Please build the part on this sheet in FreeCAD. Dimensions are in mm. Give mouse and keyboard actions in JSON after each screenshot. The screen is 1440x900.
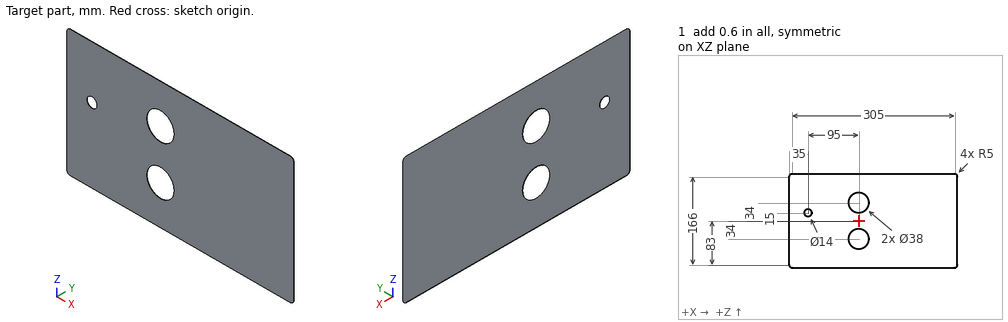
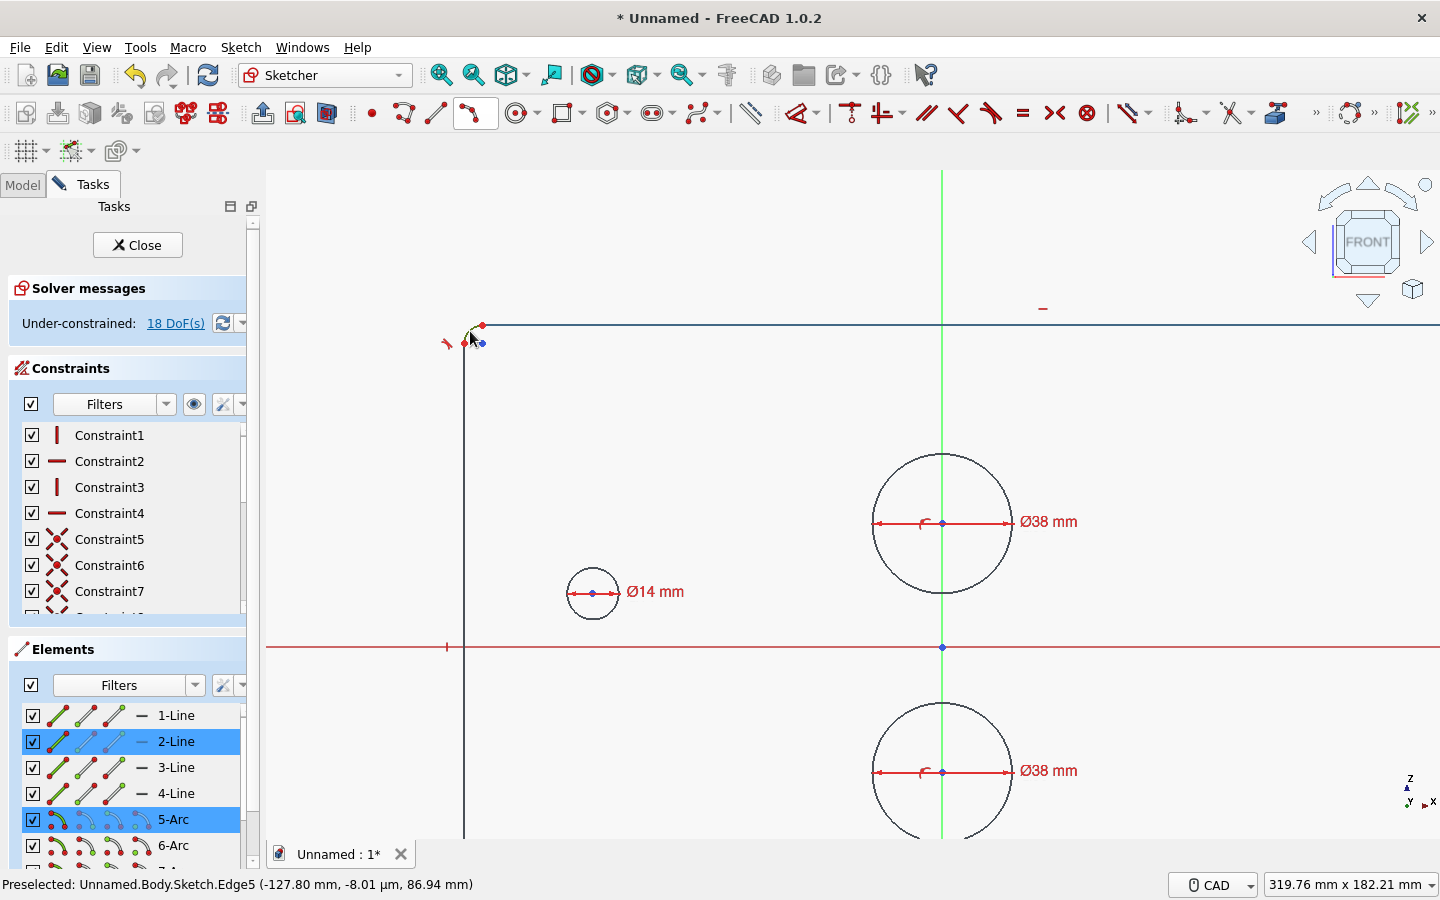
{"action": "left_click", "coordinate": [992, 114]}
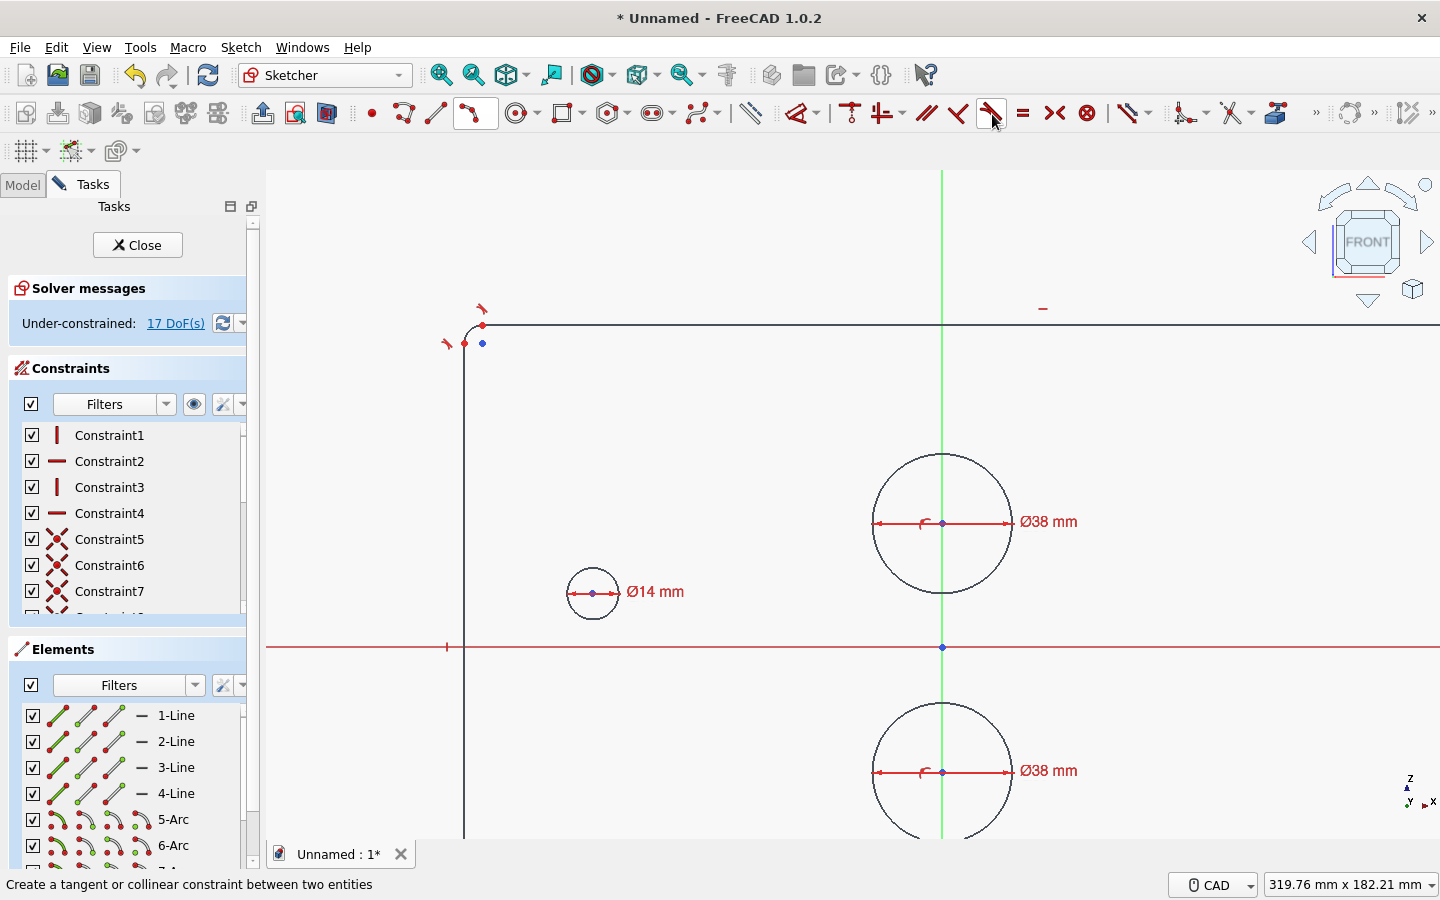
{"action": "left_click", "coordinate": [819, 325]}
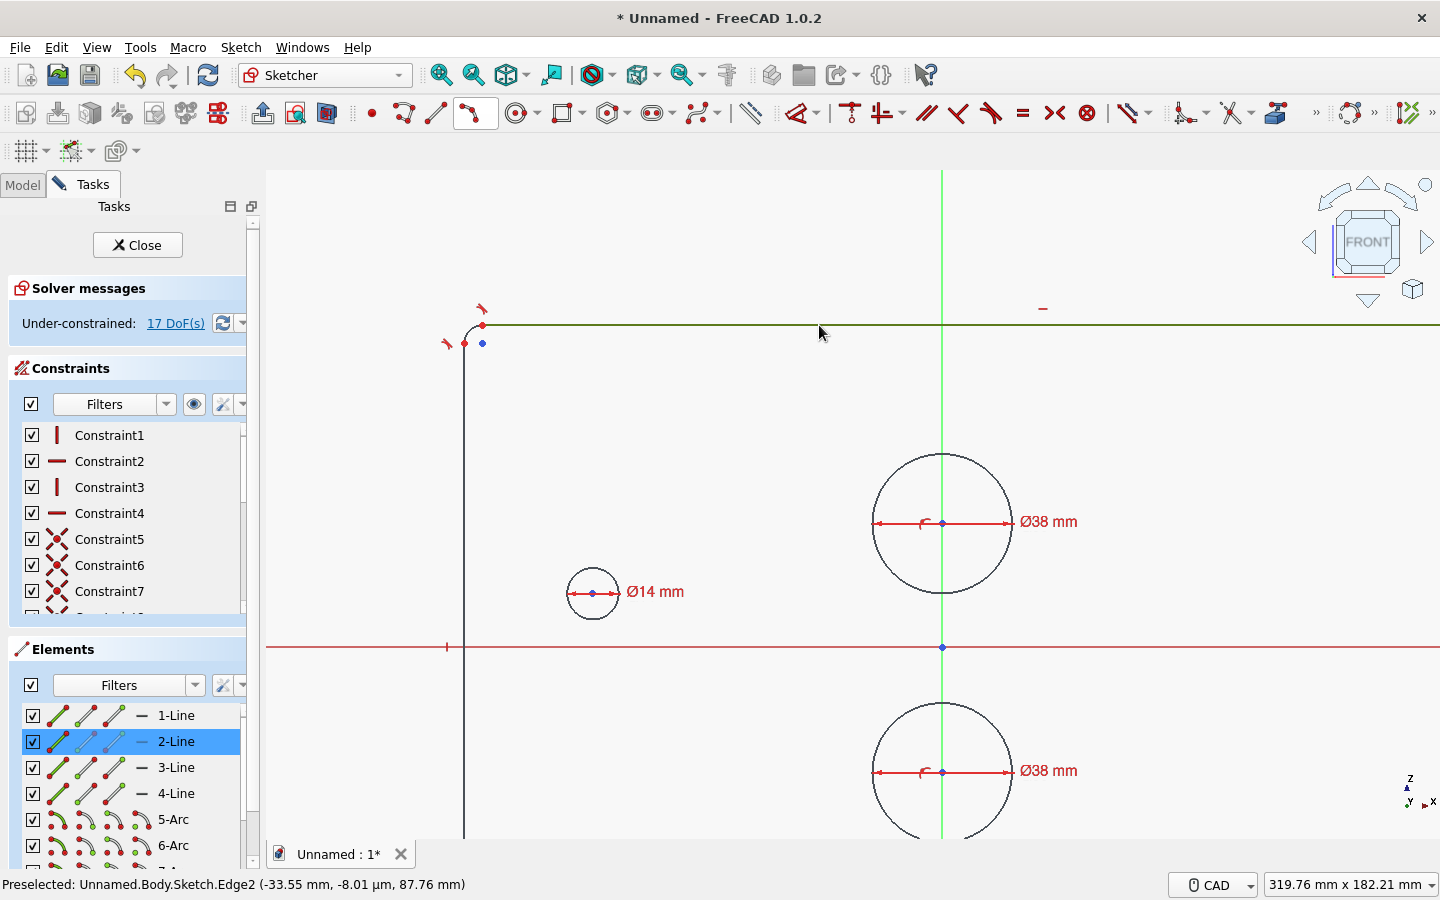
{"action": "scroll", "coordinate": [470, 331], "scroll_direction": "down", "scroll_amount": 3}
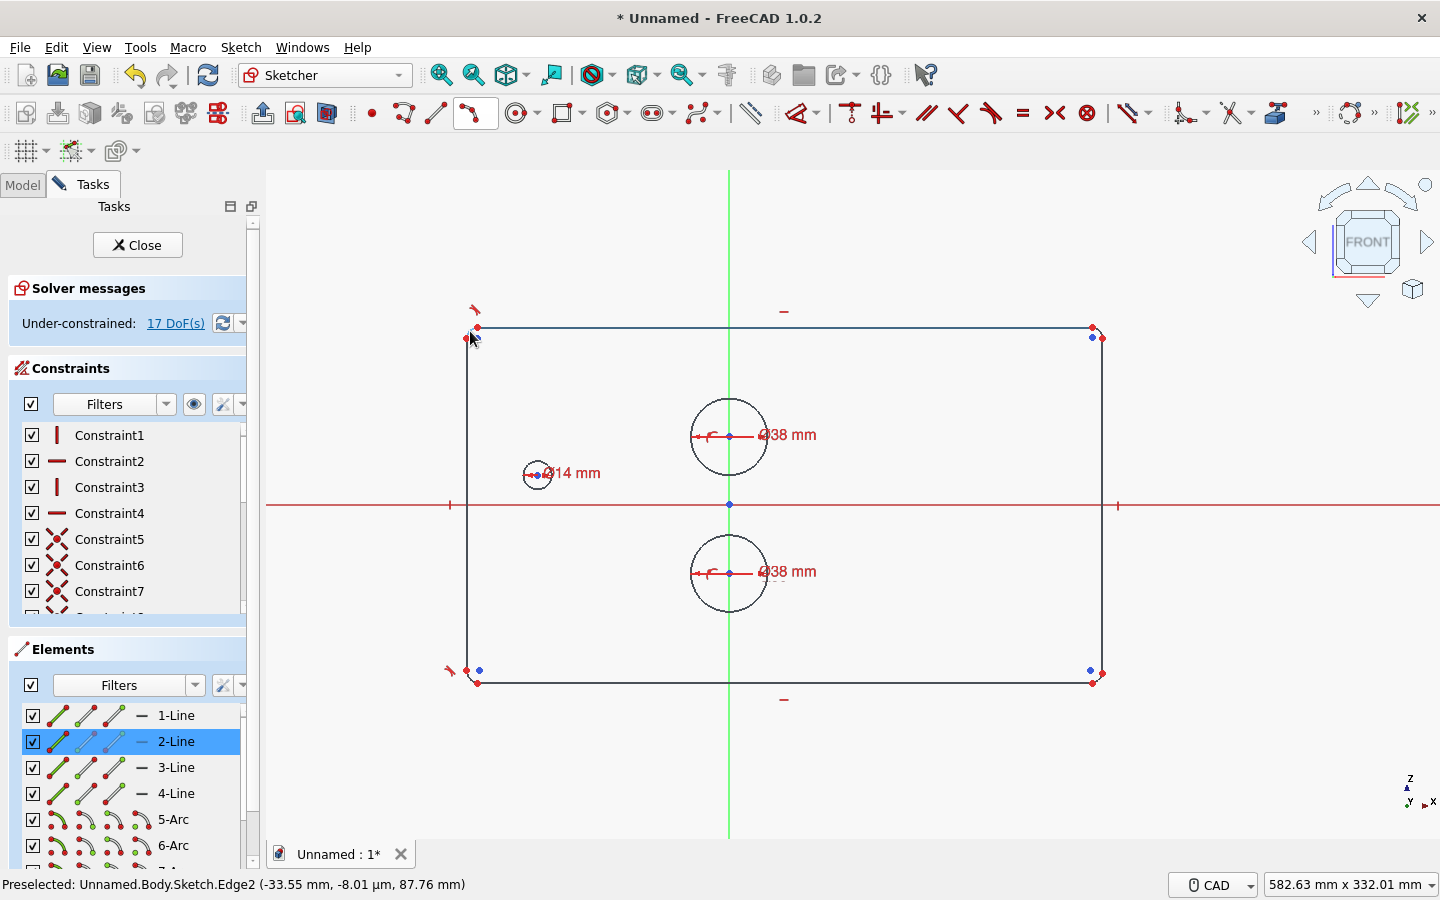
{"action": "scroll", "coordinate": [1099, 331], "scroll_direction": "up", "scroll_amount": 3}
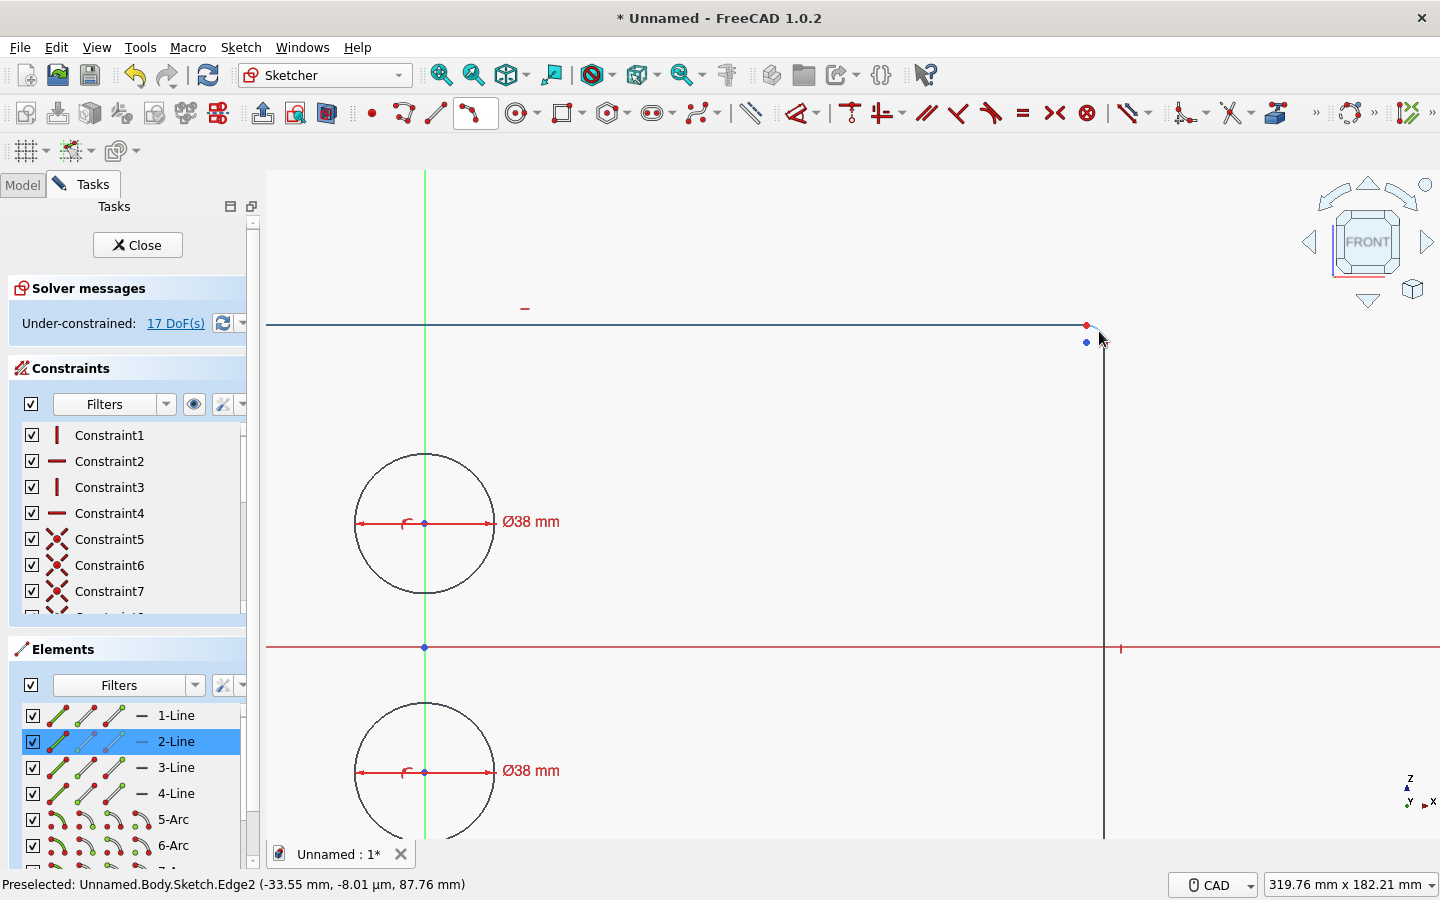
{"action": "left_click", "coordinate": [1099, 330]}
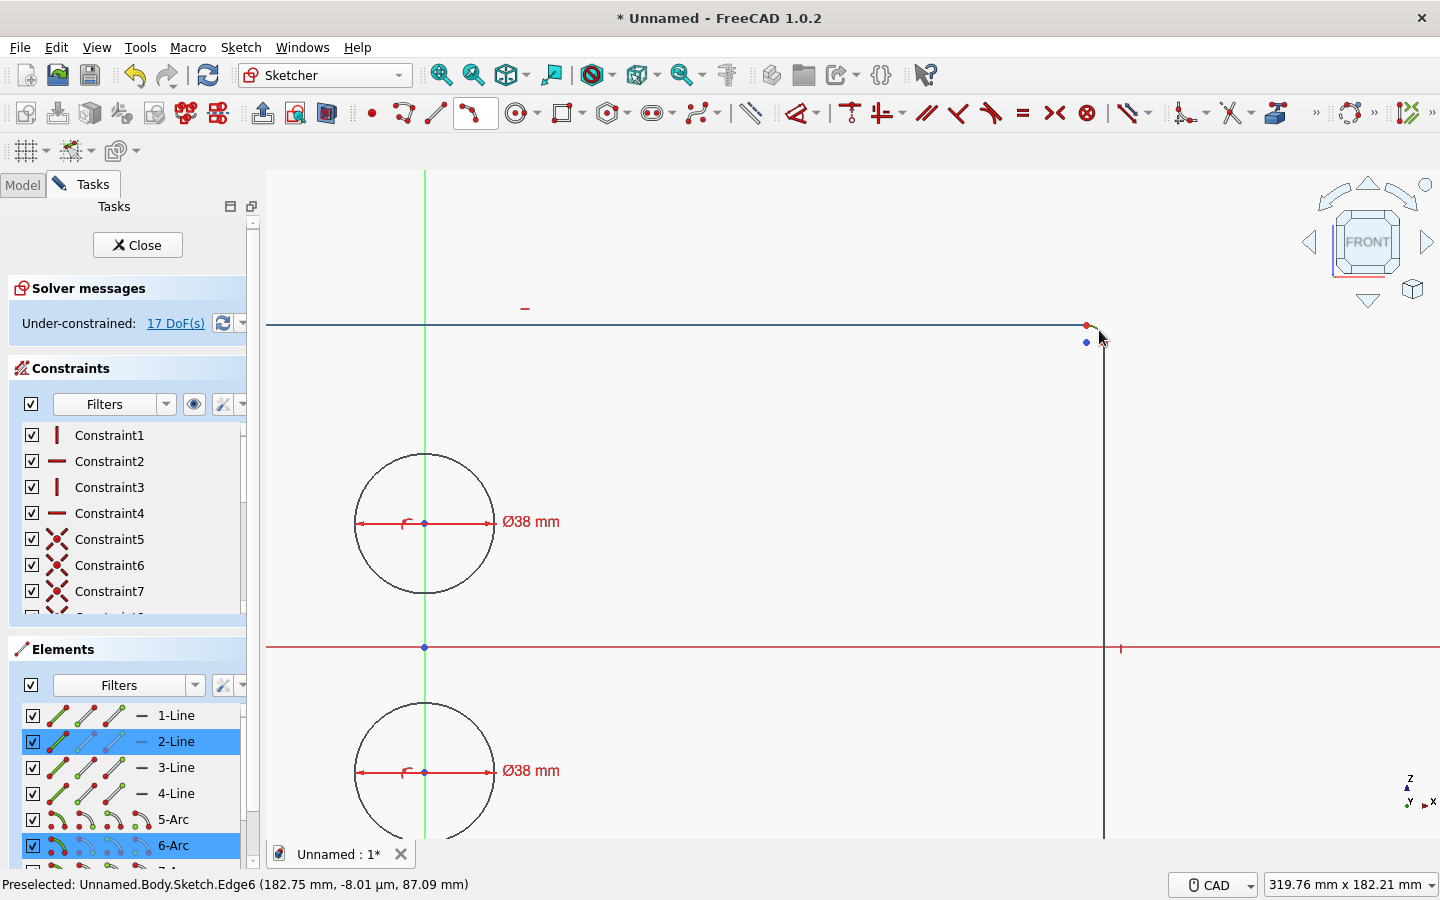
{"action": "left_click", "coordinate": [992, 114]}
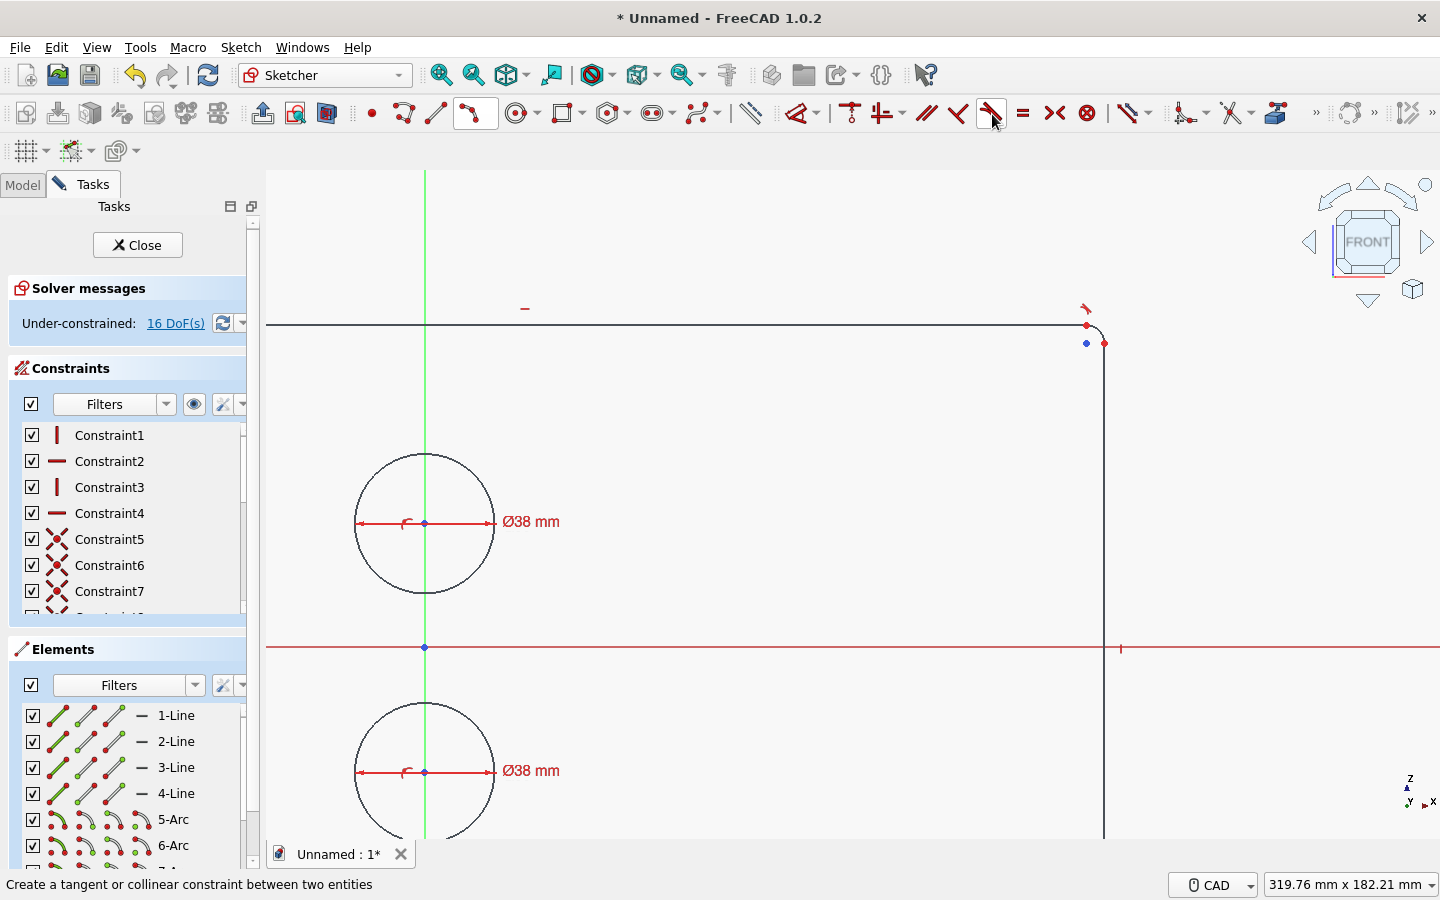
{"action": "left_click", "coordinate": [1104, 527]}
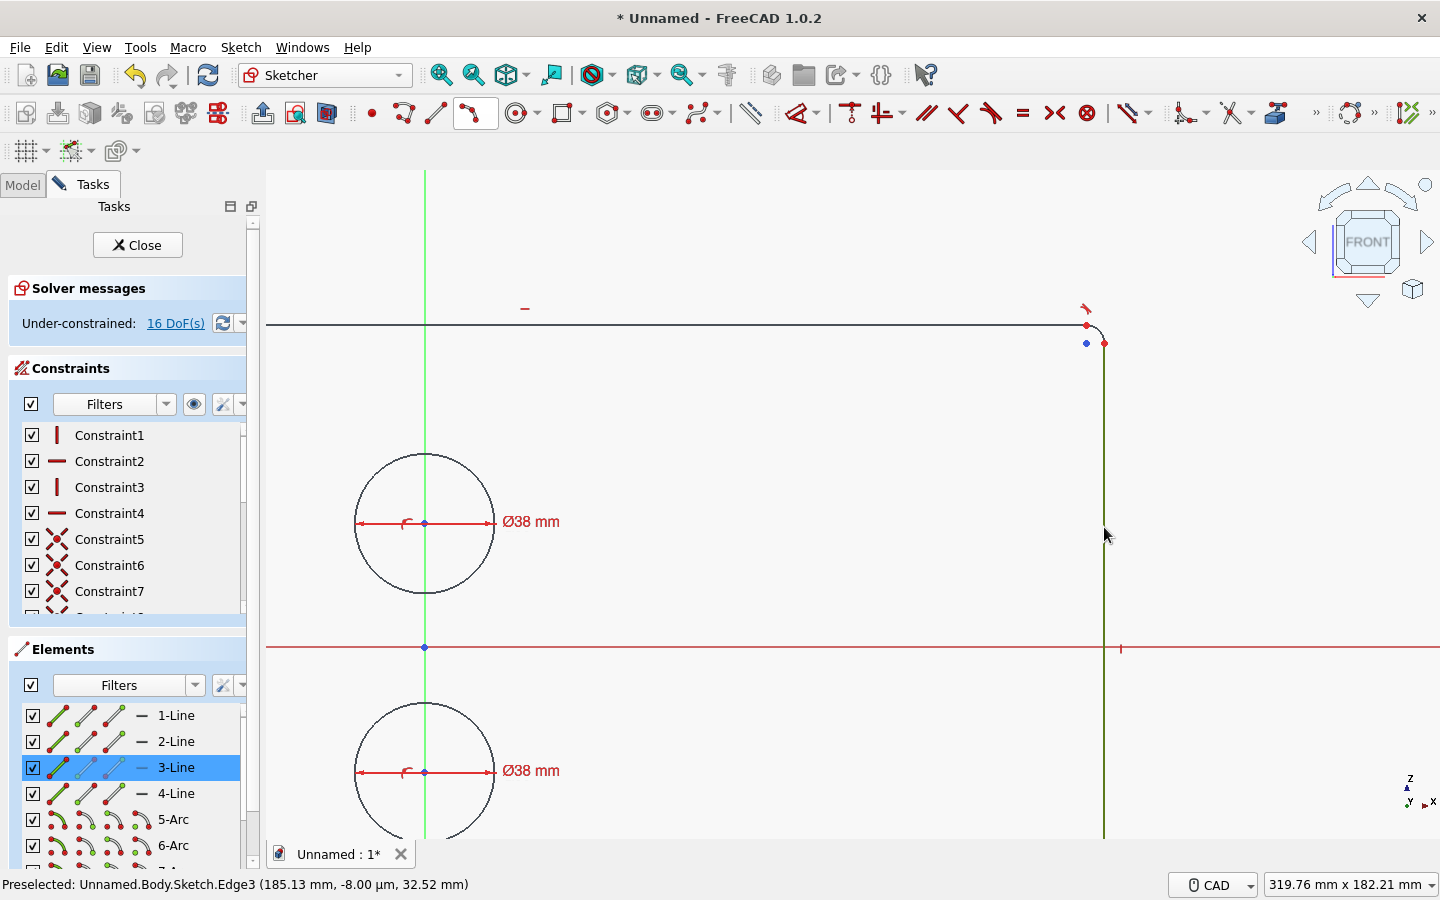
{"action": "left_click", "coordinate": [1099, 331]}